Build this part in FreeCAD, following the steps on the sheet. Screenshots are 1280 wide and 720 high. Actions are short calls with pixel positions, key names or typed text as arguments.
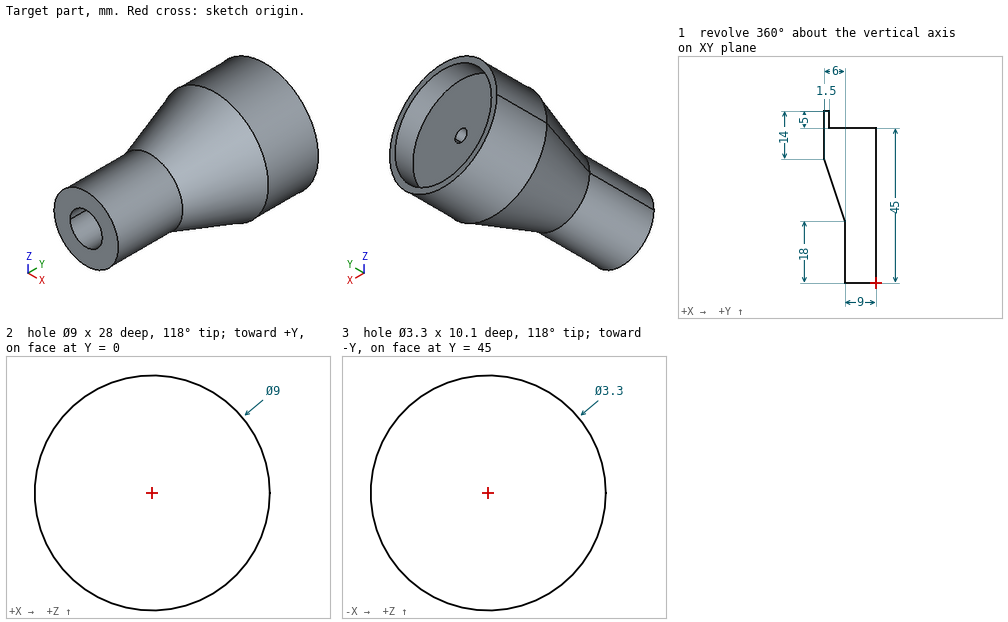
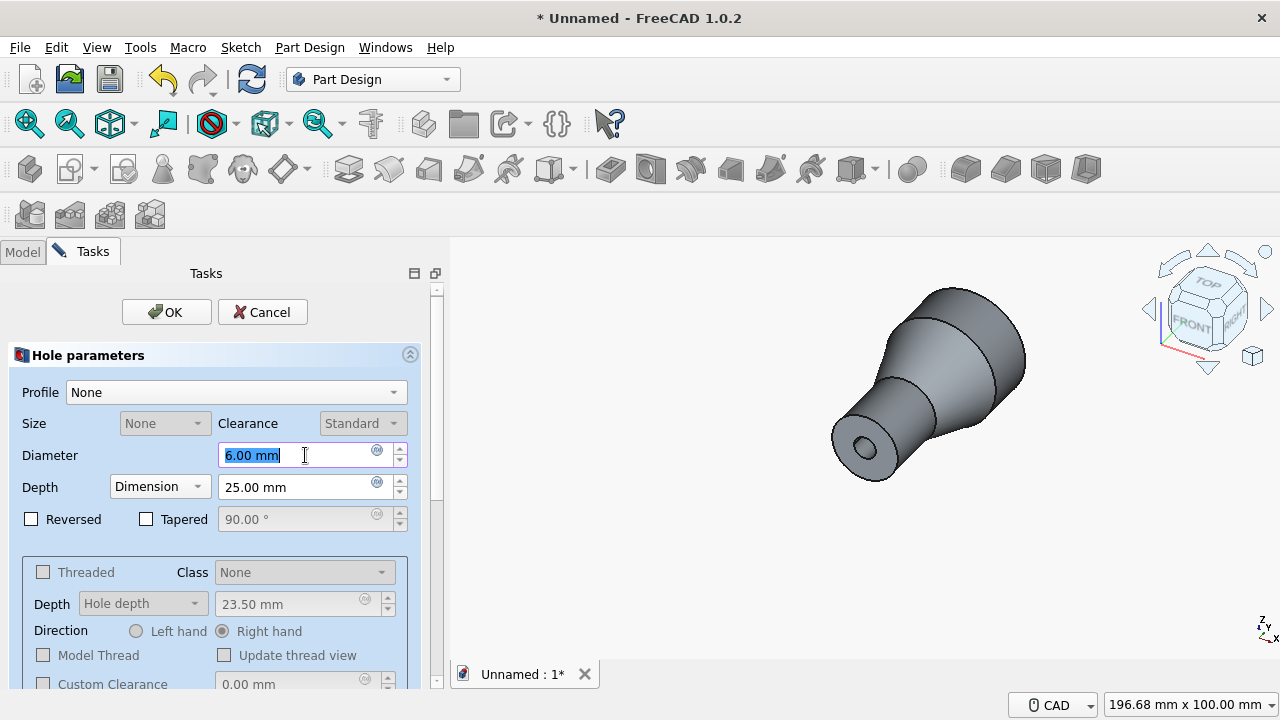
text(9)
key(Tab)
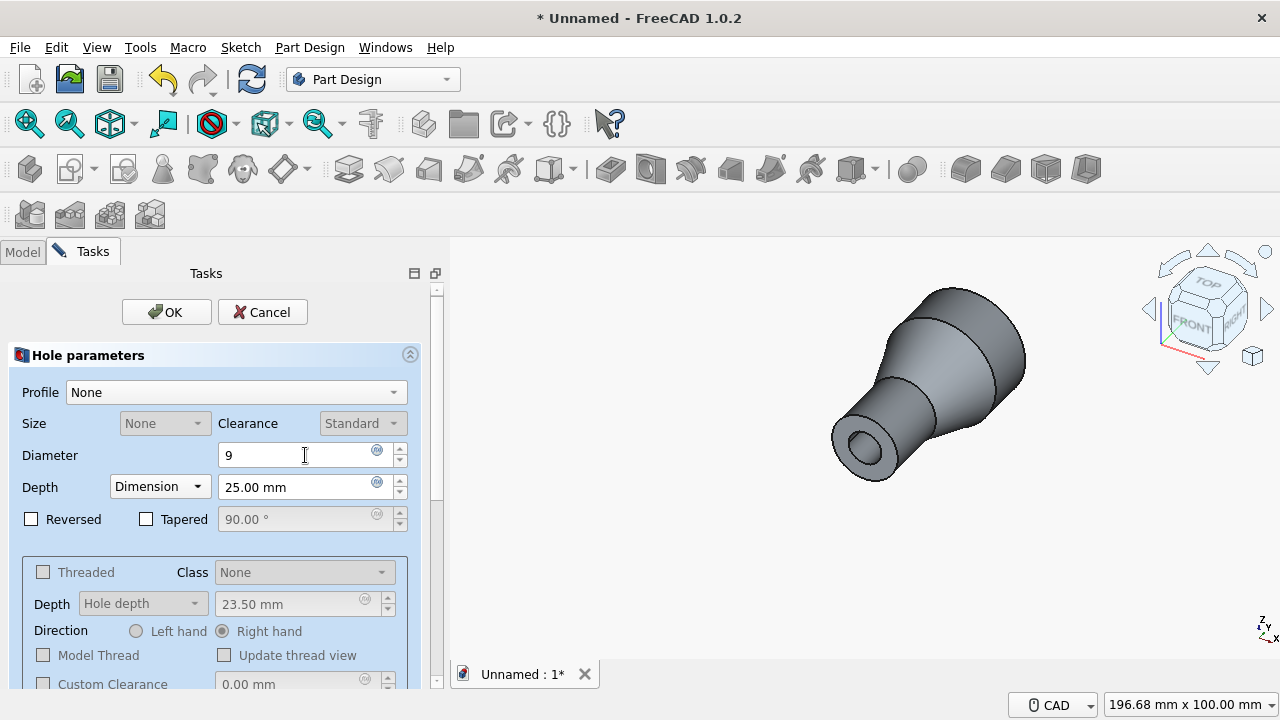
triple_click(305, 487)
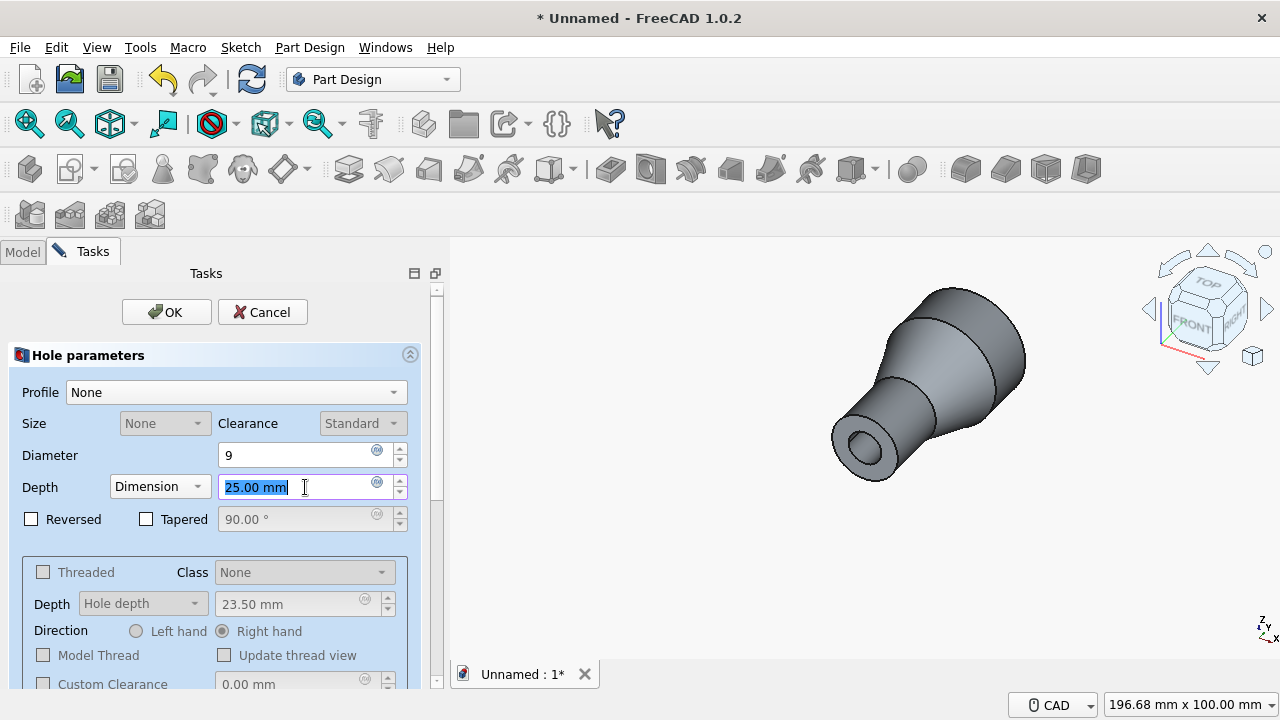
text(28)
key(Tab)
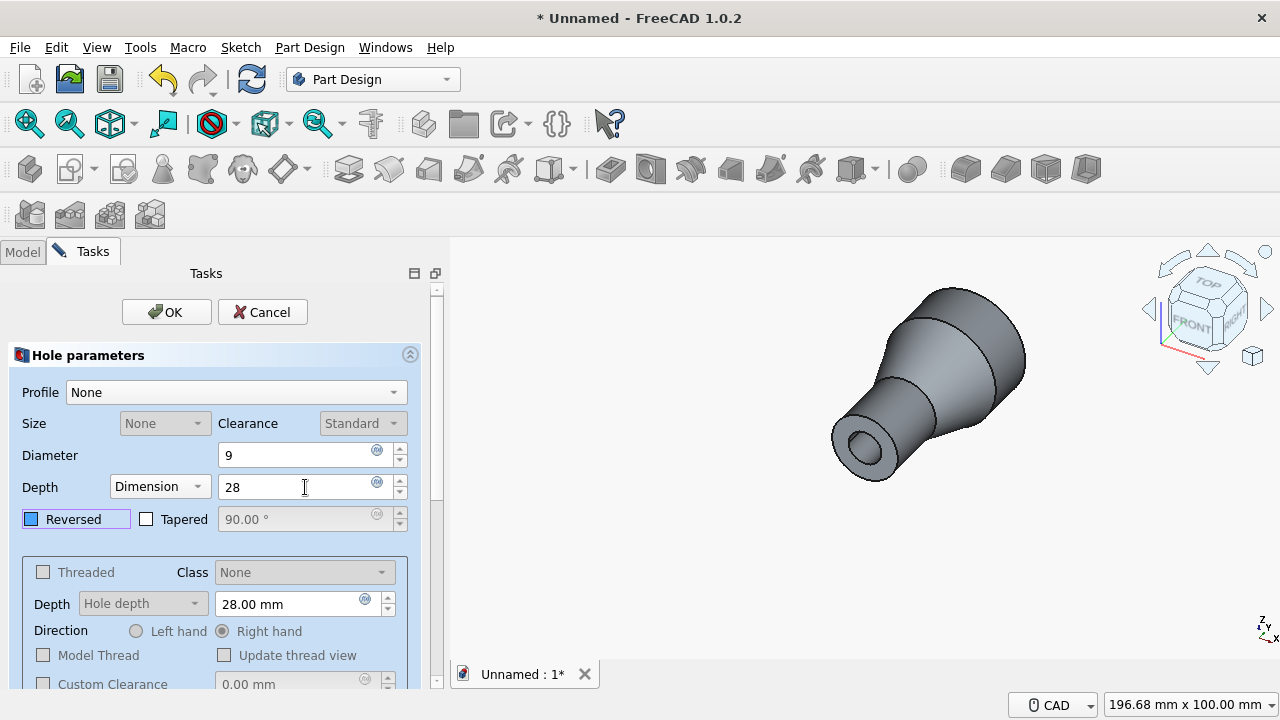
click(167, 312)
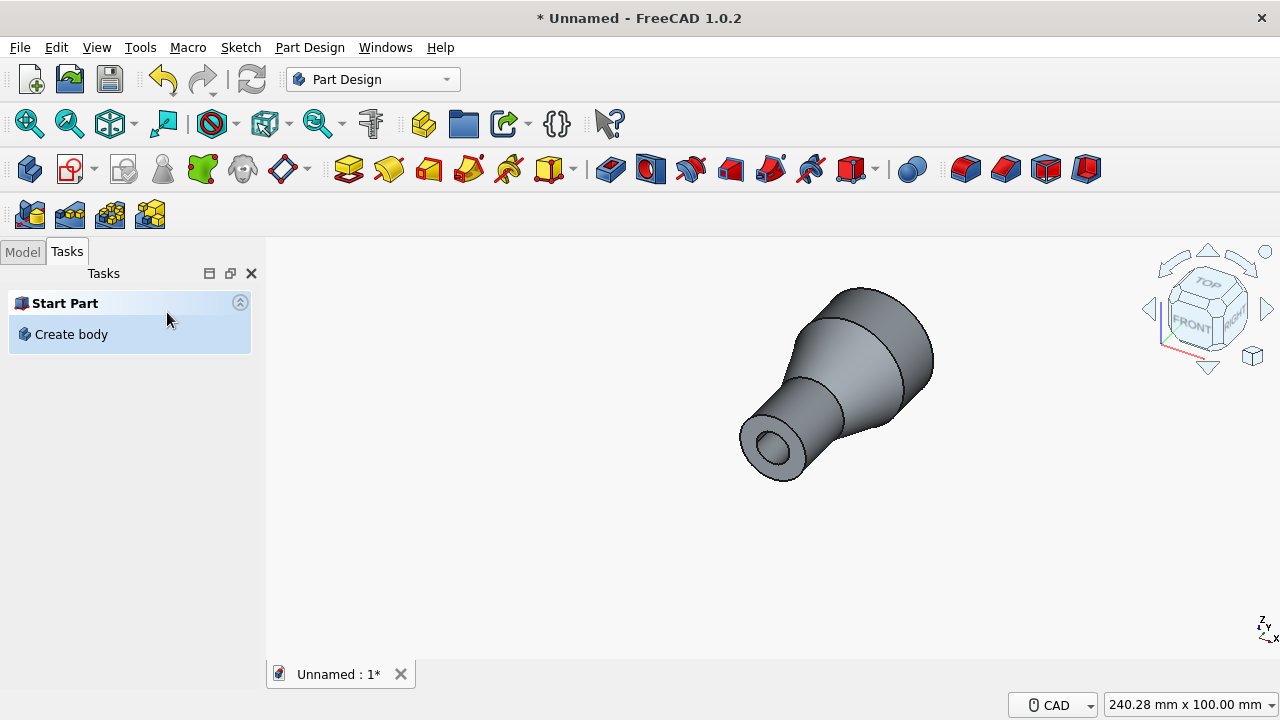
key(4)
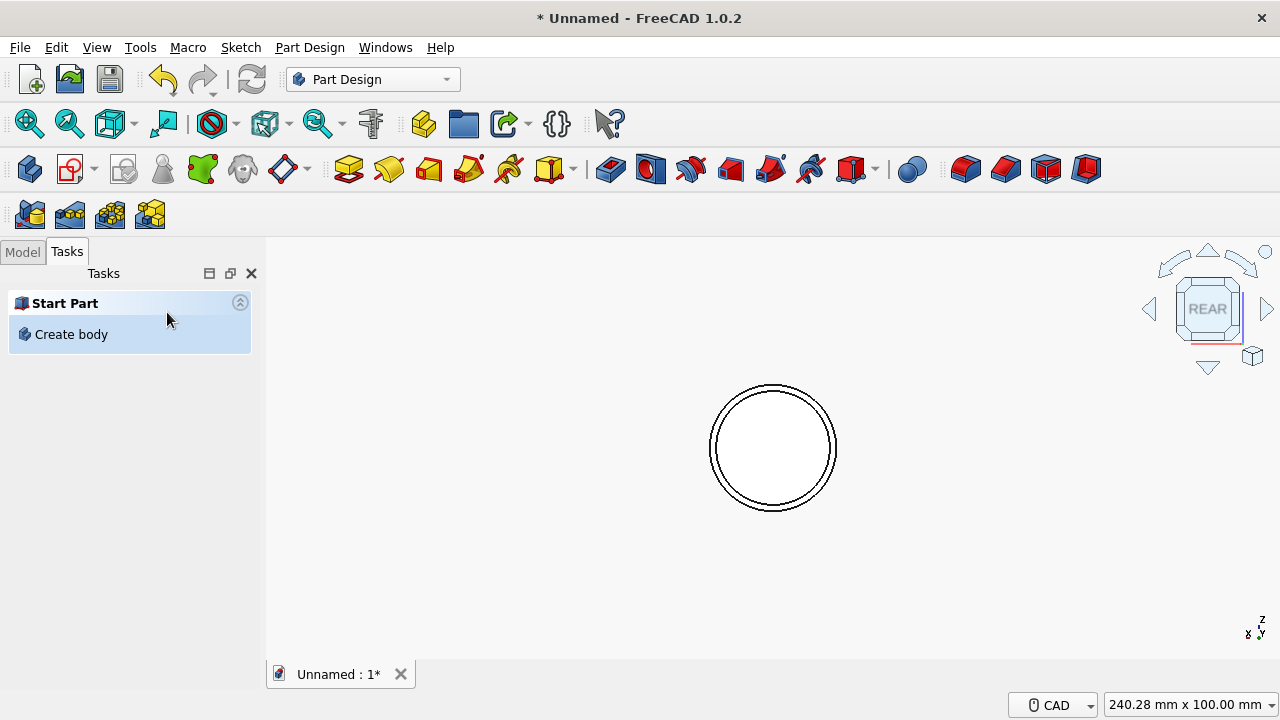
click(30, 124)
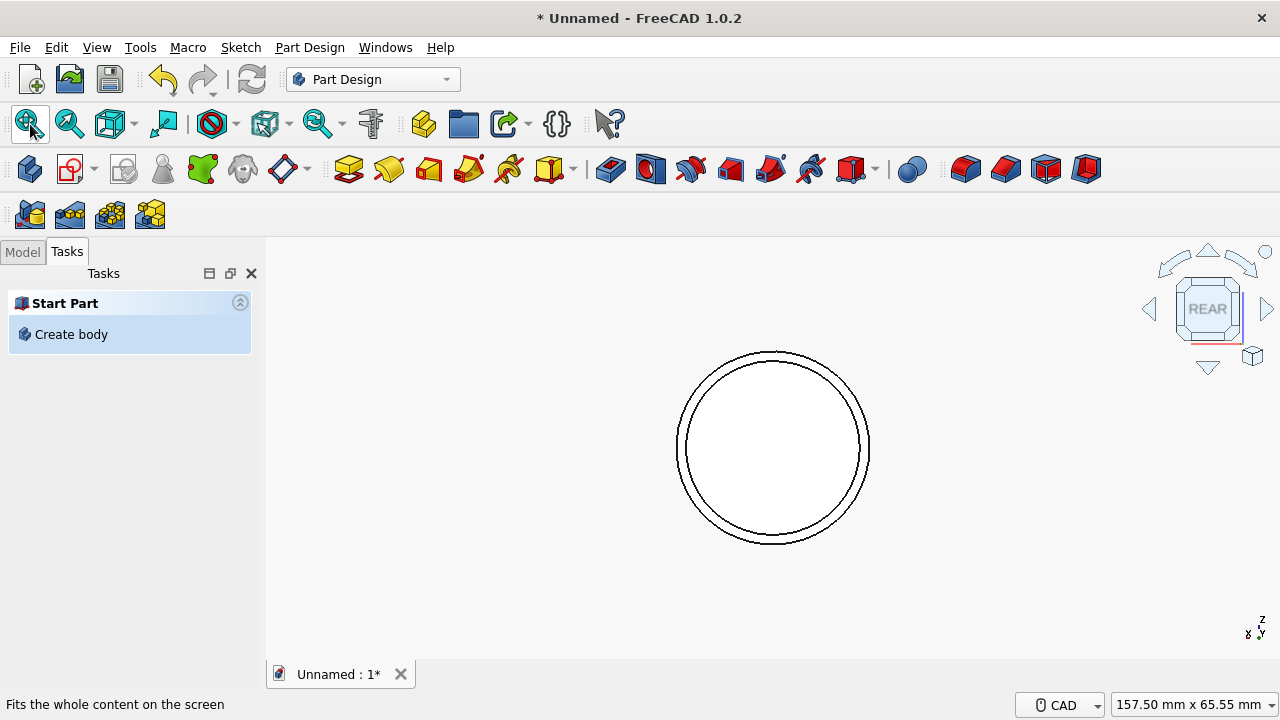
click(773, 447)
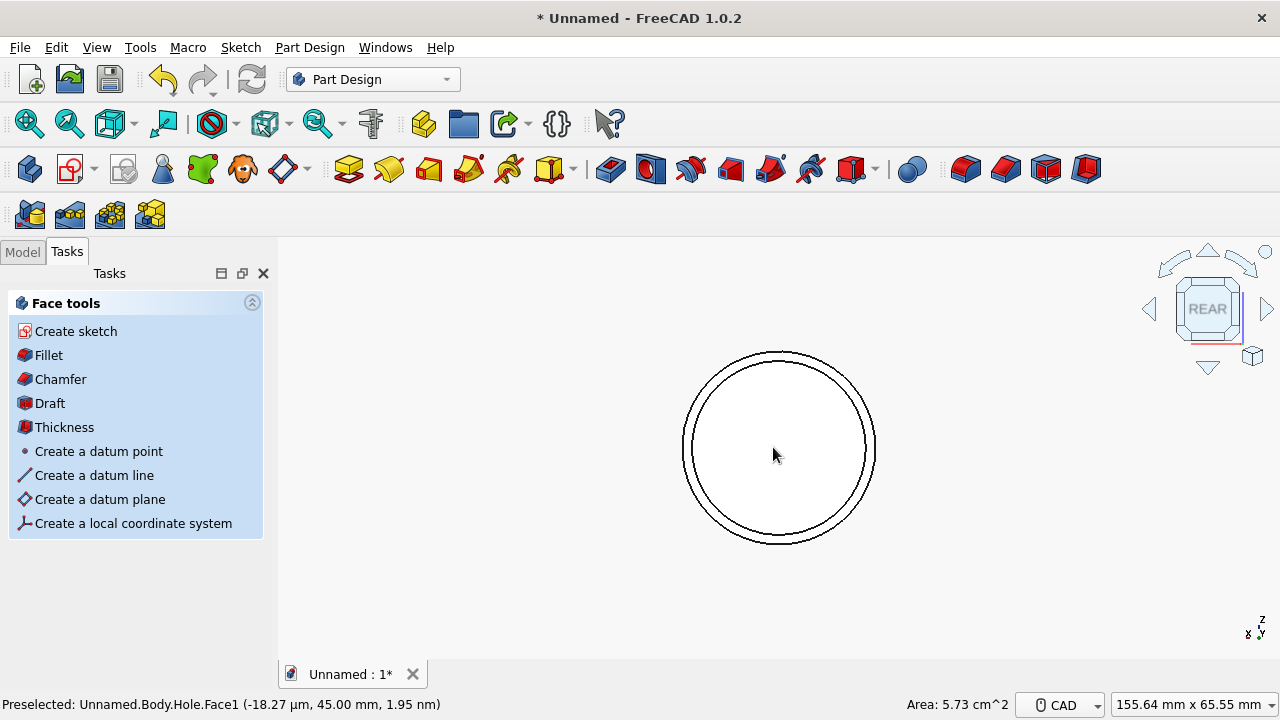
click(70, 170)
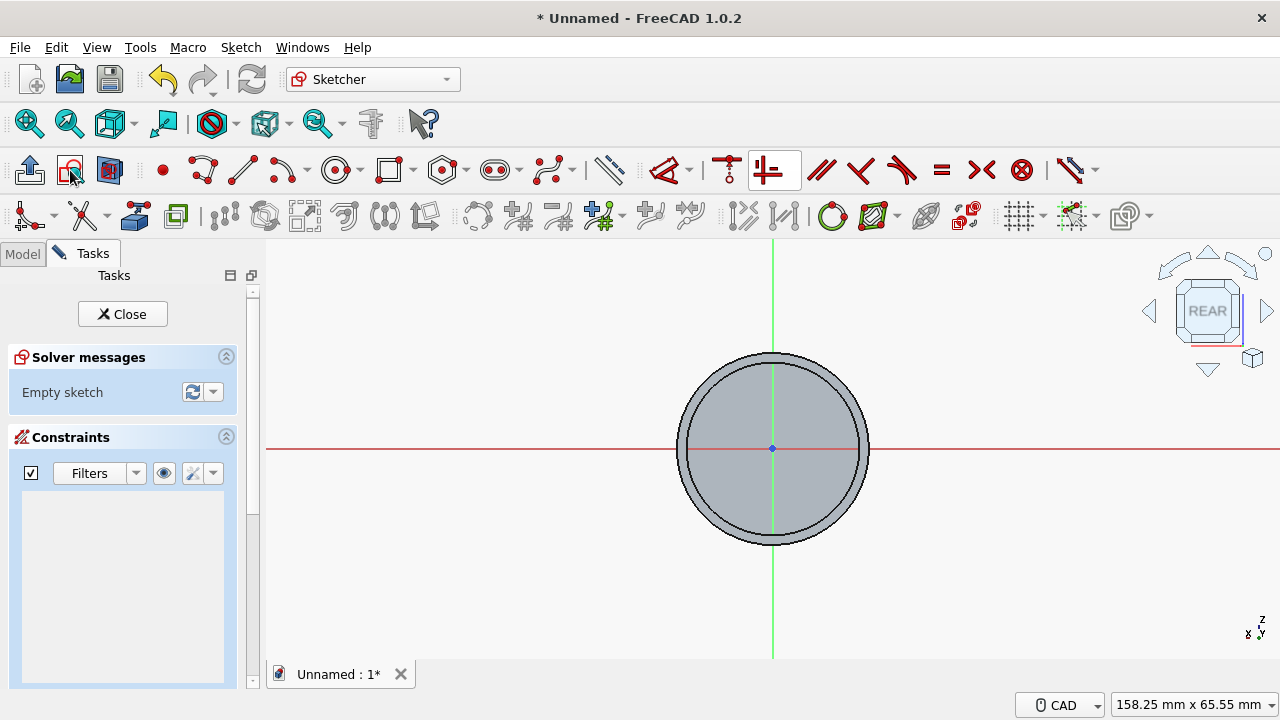
click(110, 170)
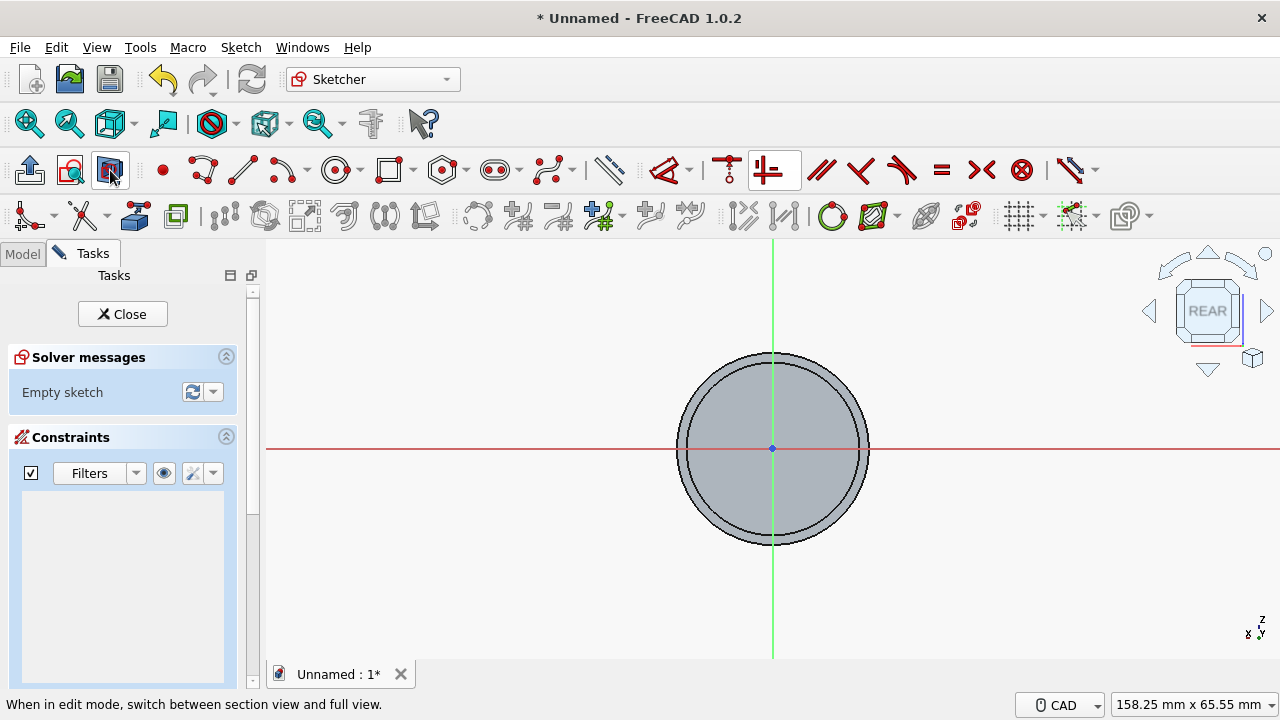
scroll(780, 449, up, 12)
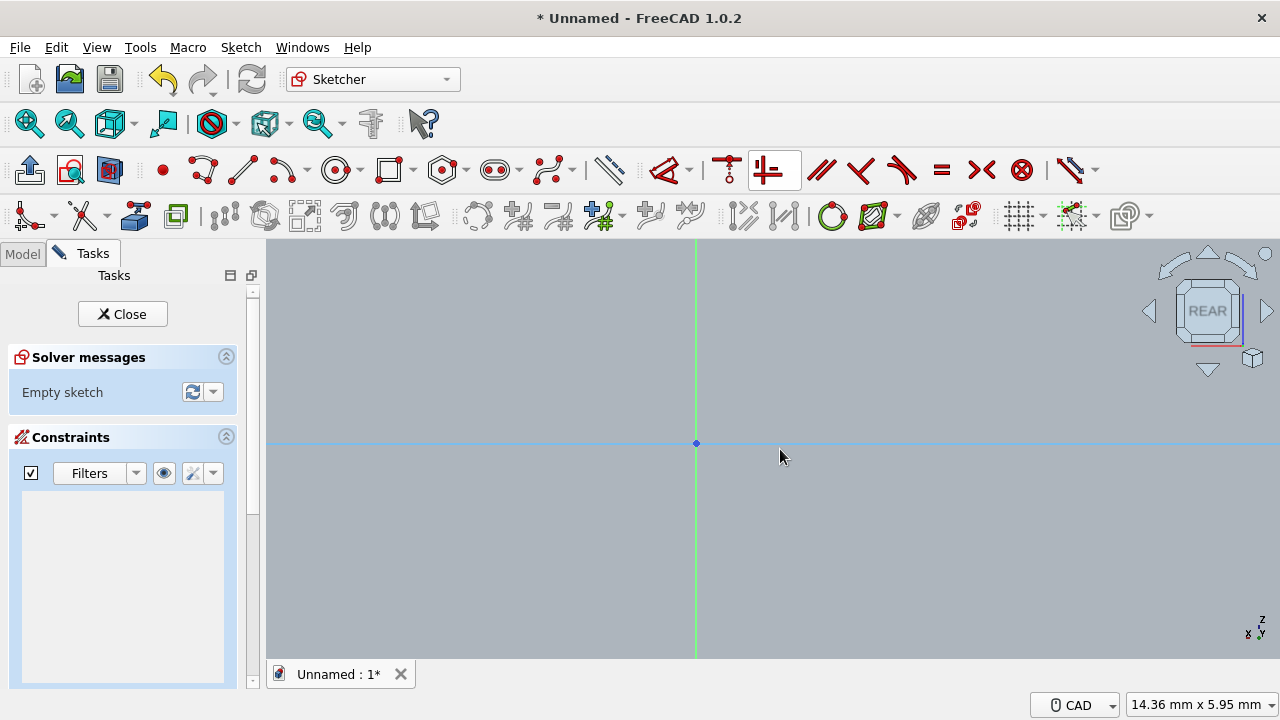
click(336, 170)